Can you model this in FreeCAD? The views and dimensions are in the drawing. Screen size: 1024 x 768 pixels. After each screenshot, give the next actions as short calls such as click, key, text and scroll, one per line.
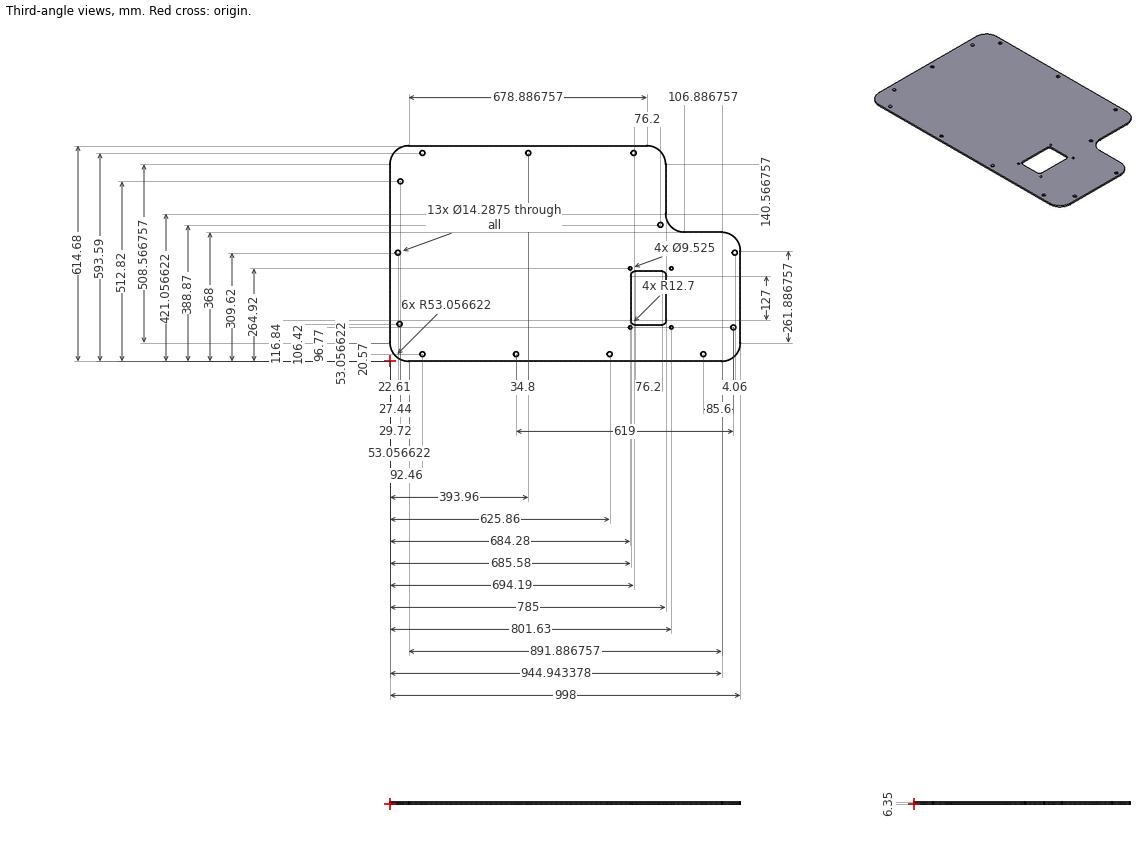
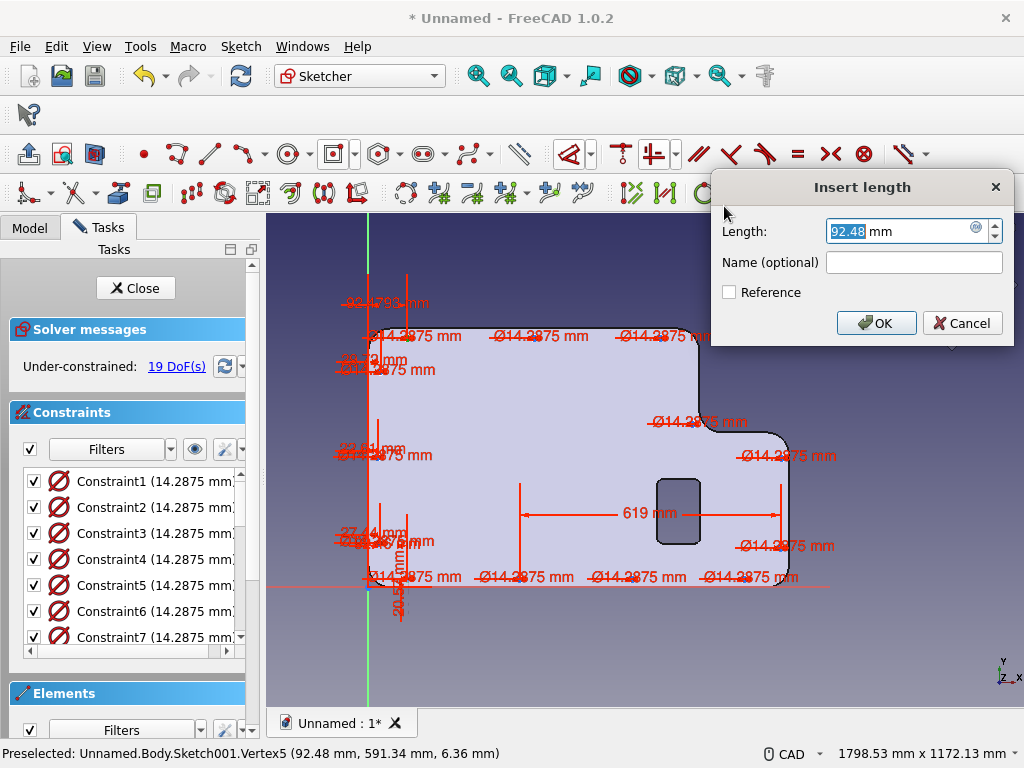
text(92.46)
key(Return)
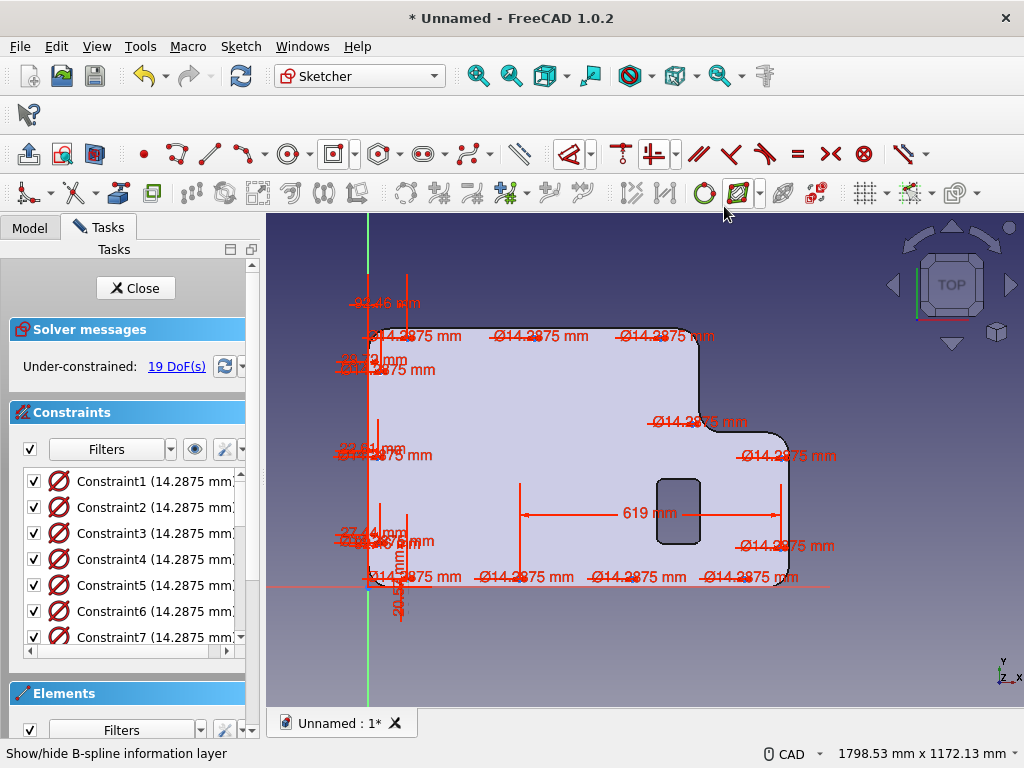
scroll(520, 579, up, 8)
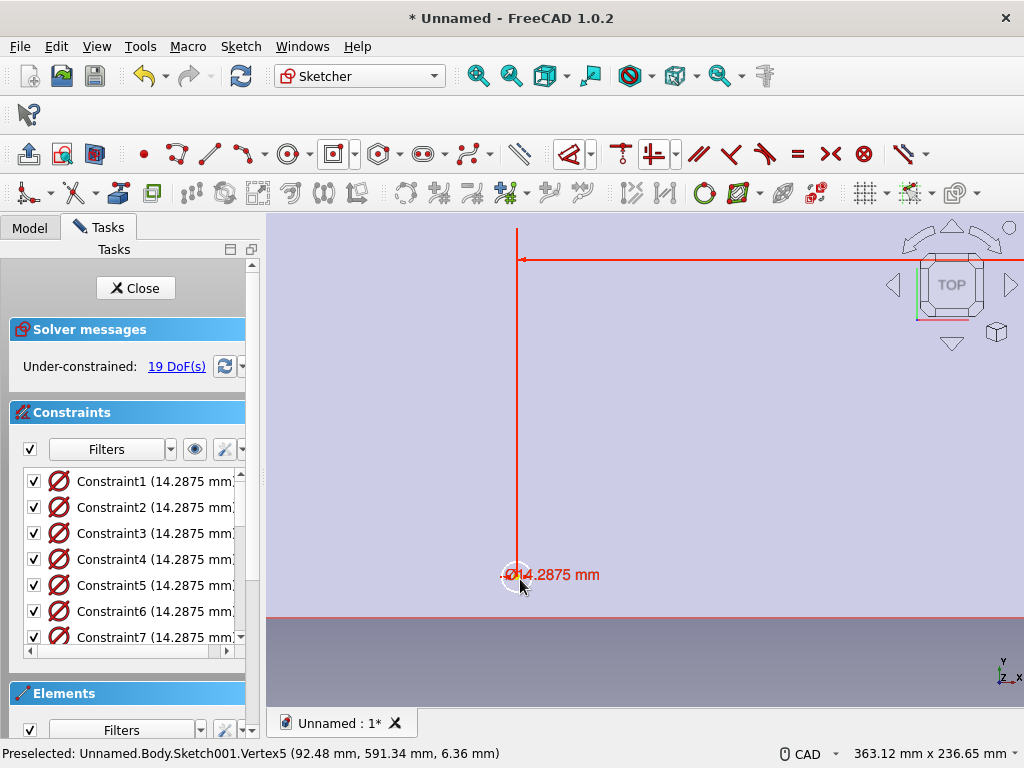
click(517, 577)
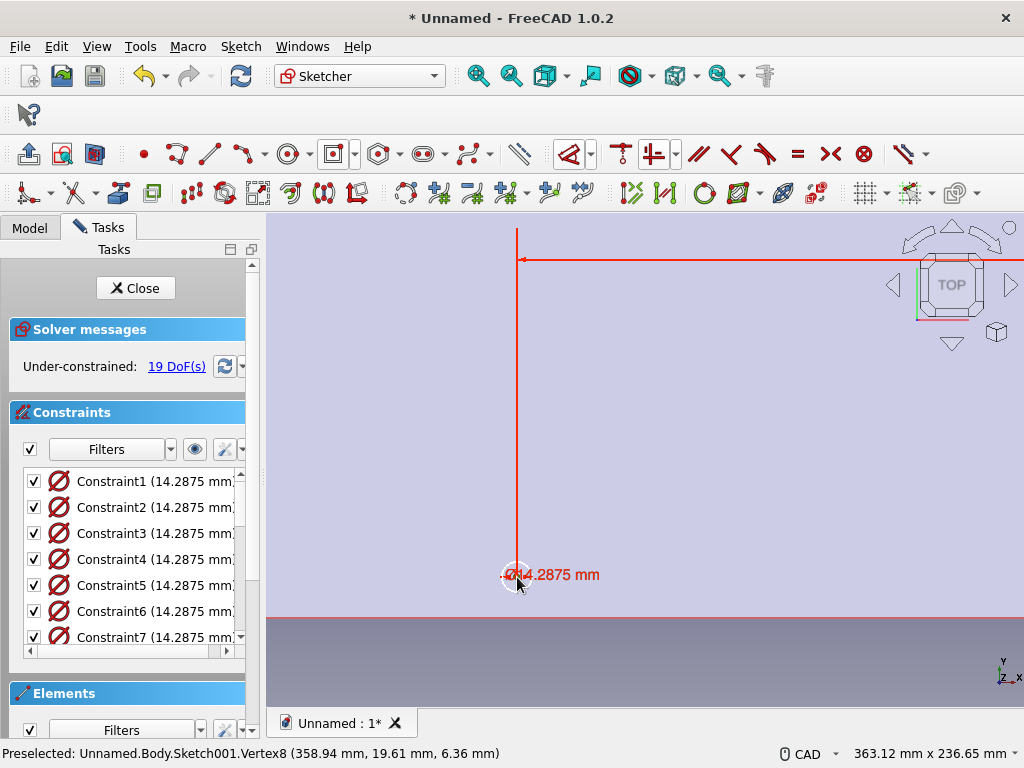
key(i)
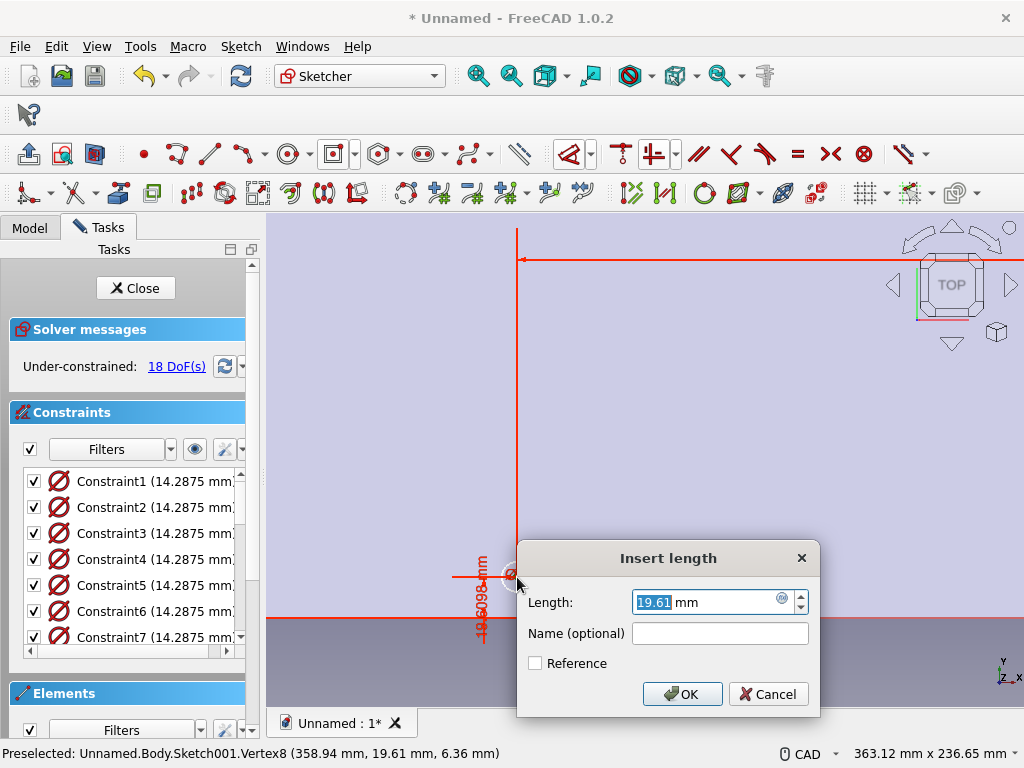
text(20.57)
key(Return)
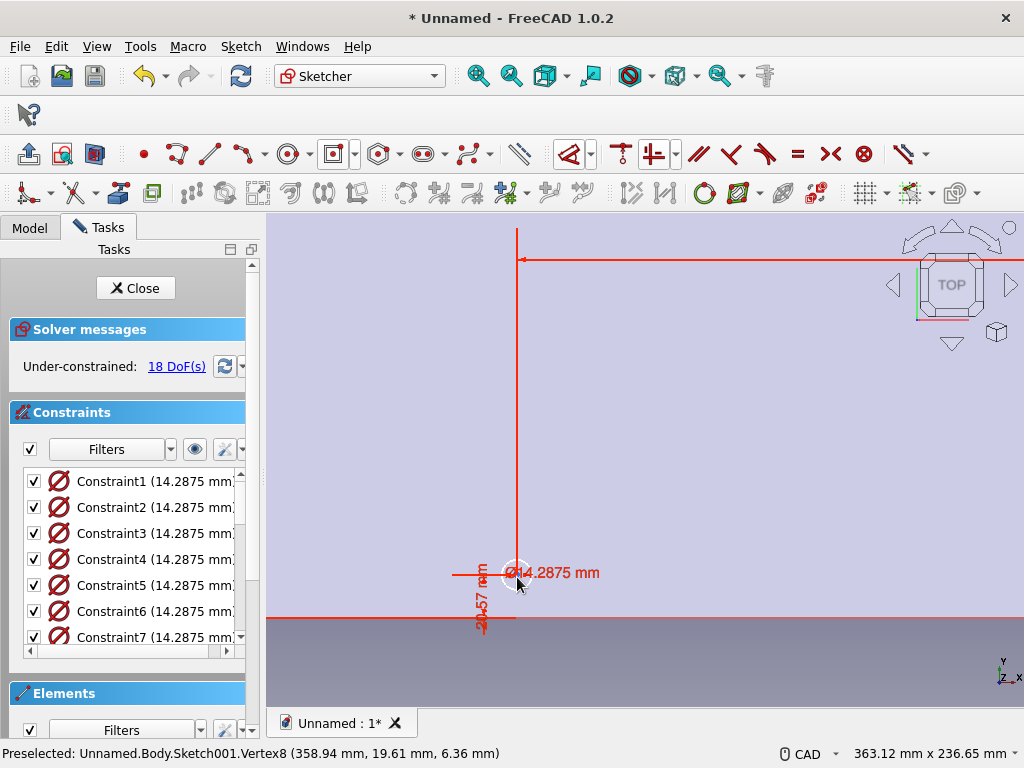
scroll(520, 579, down, 8)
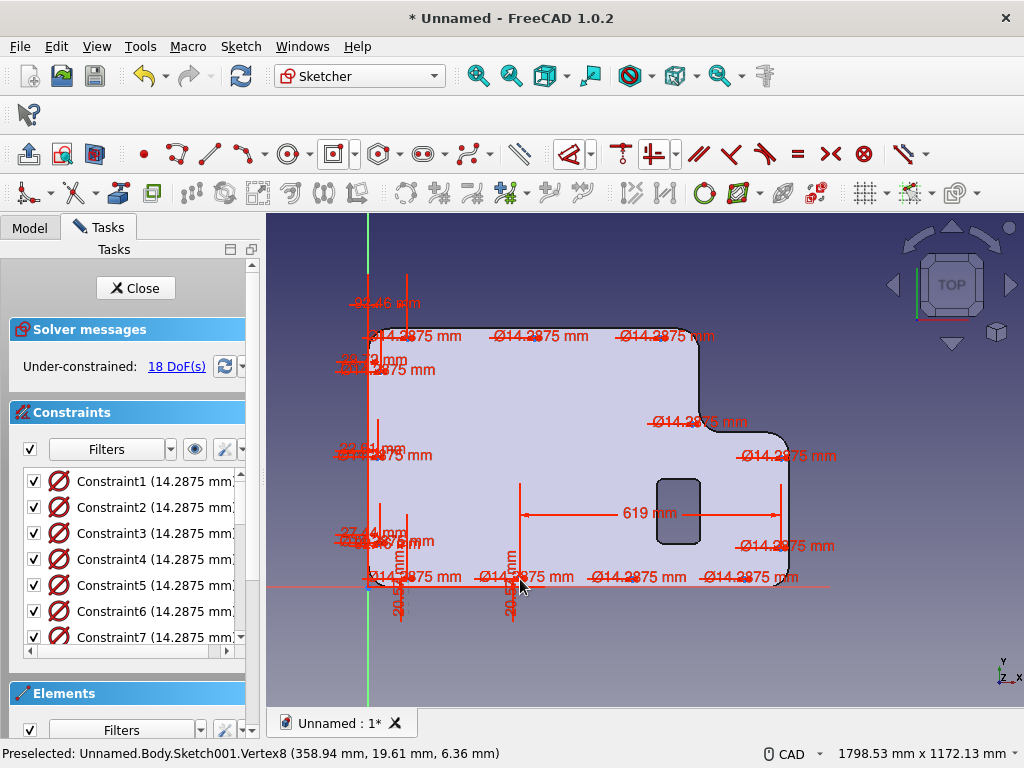
scroll(632, 579, up, 8)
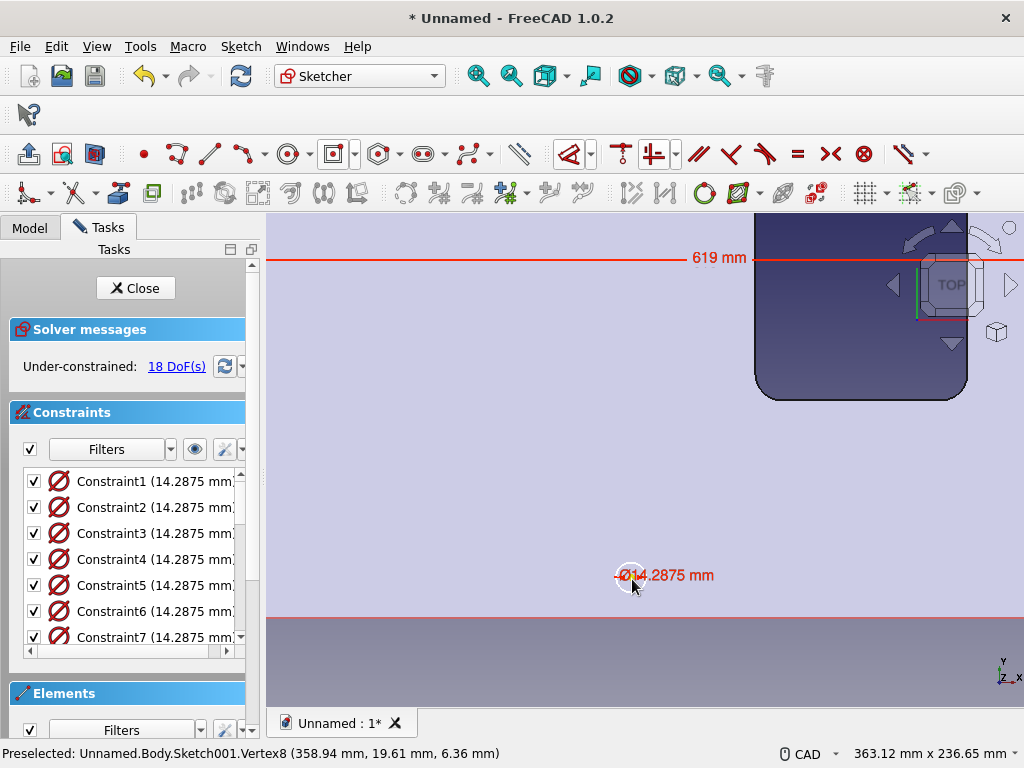
click(631, 577)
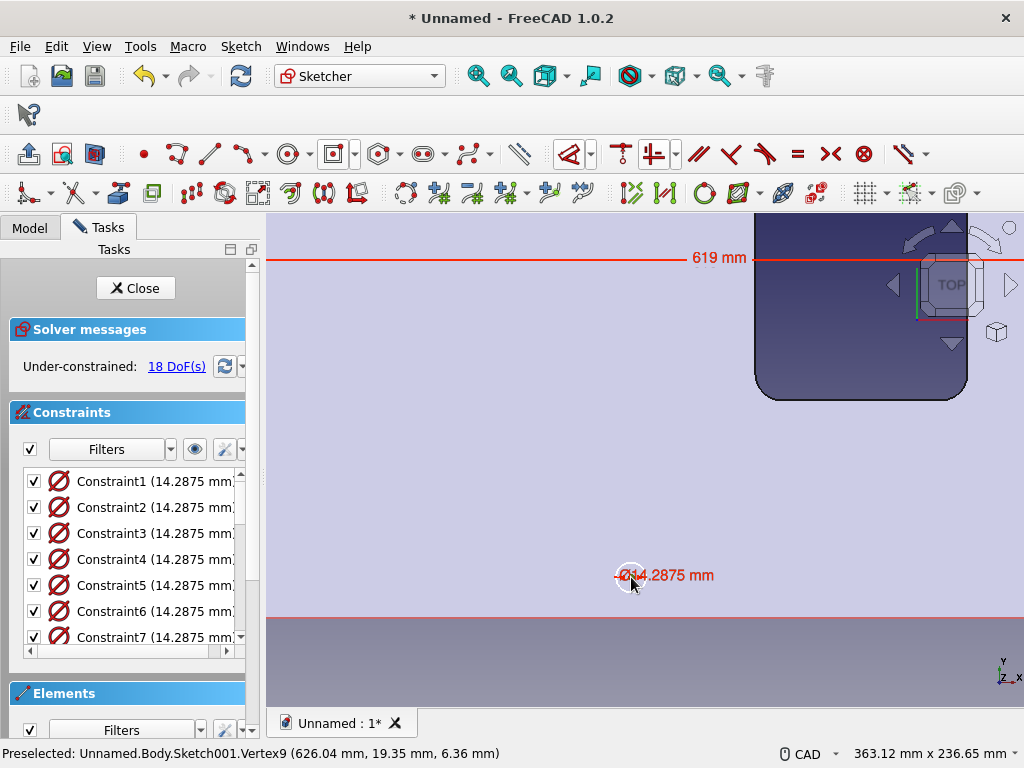
key(i)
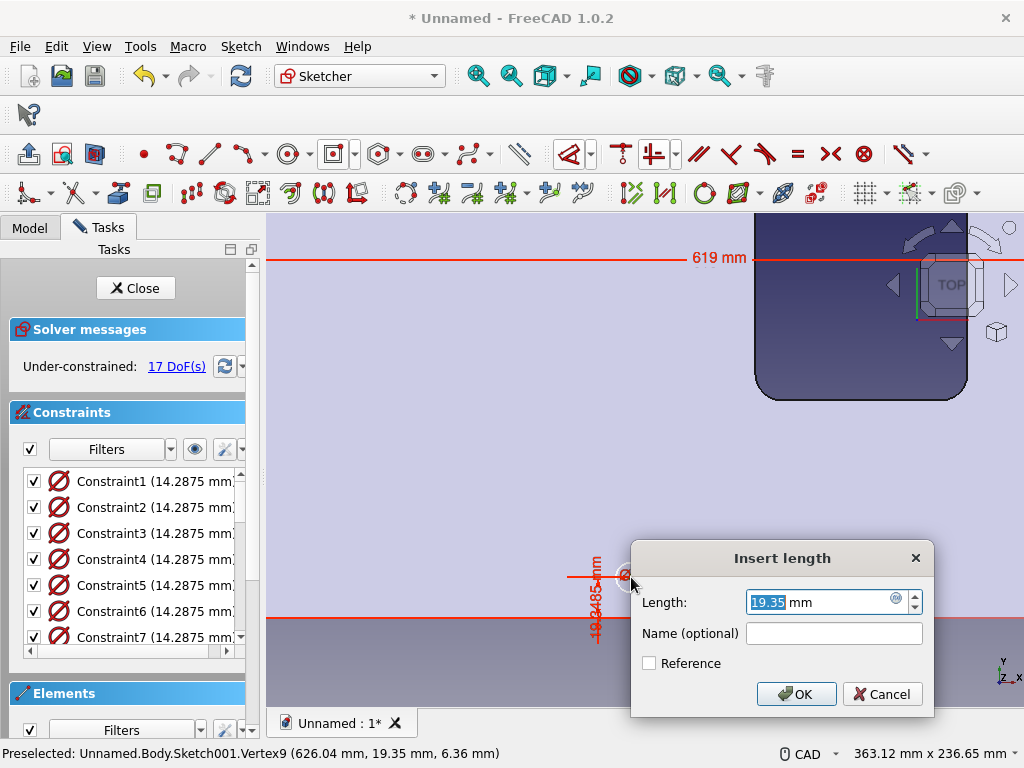
text(20.57)
key(Return)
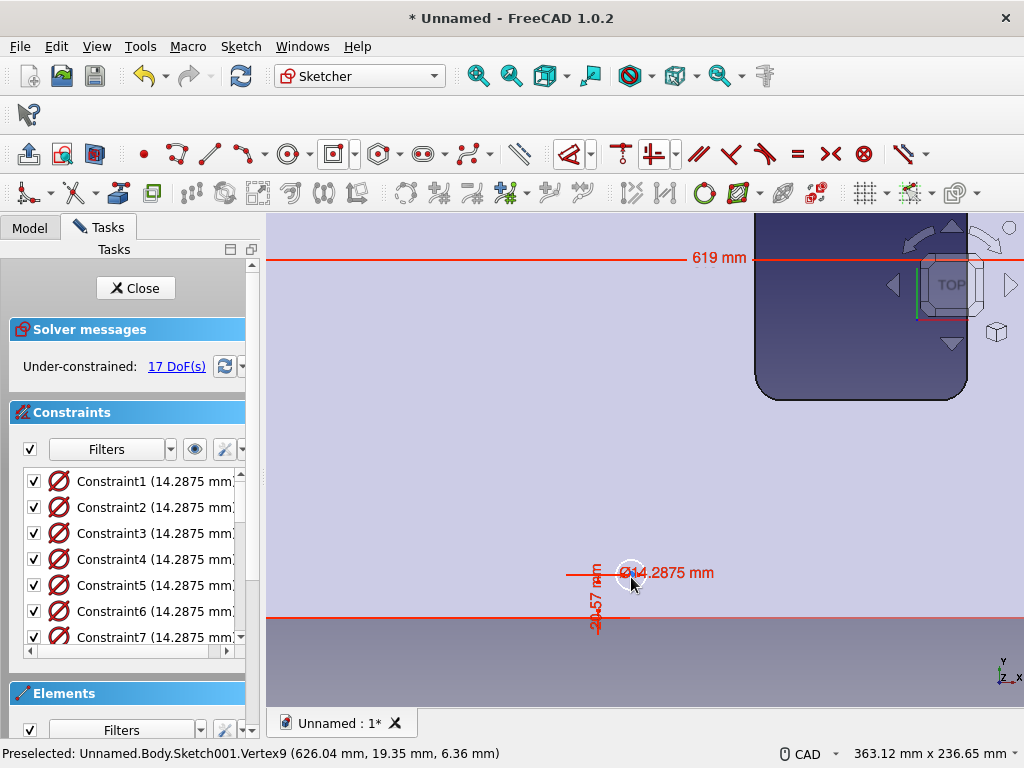
scroll(632, 579, down, 8)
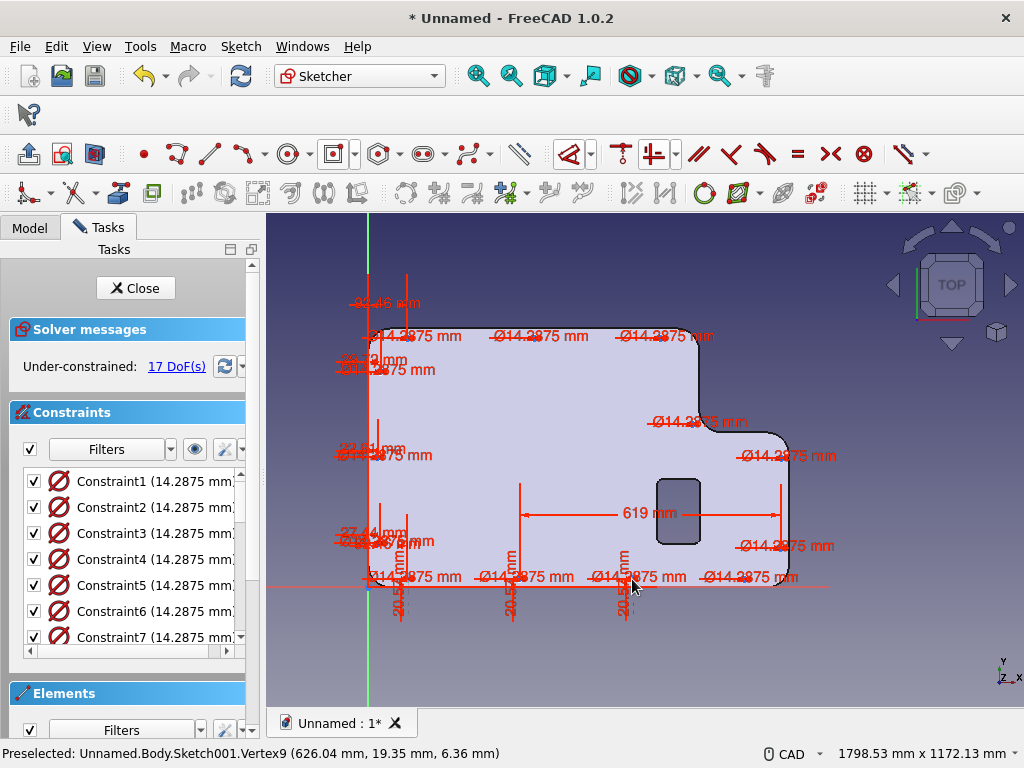
scroll(744, 579, up, 8)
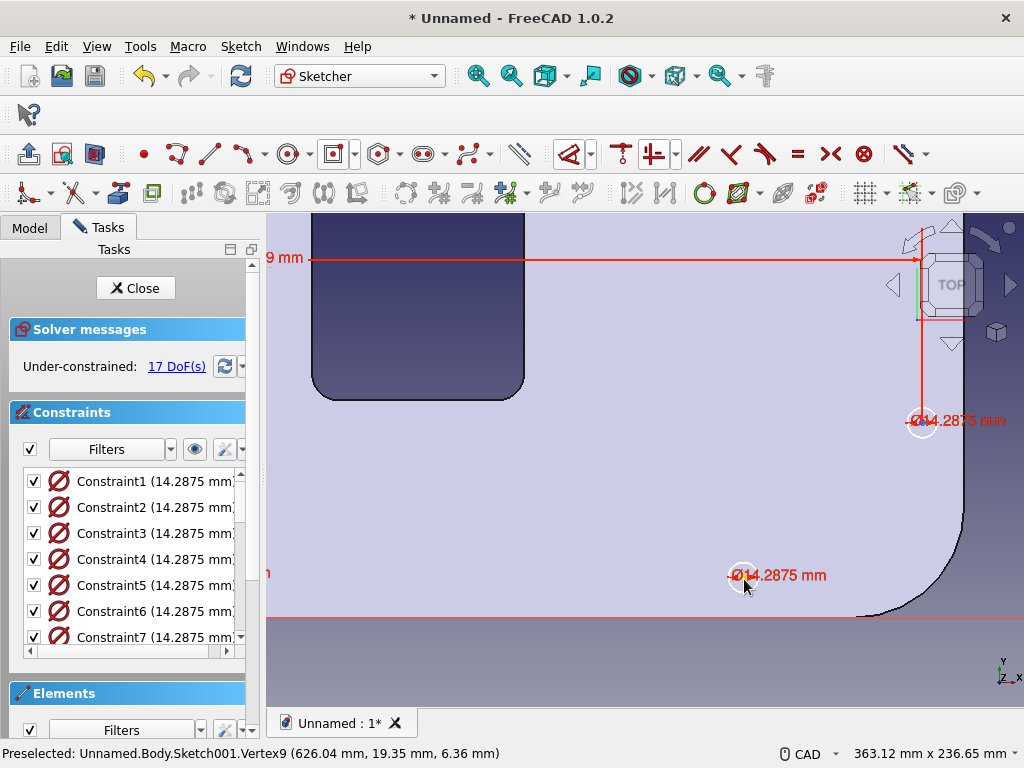
click(743, 577)